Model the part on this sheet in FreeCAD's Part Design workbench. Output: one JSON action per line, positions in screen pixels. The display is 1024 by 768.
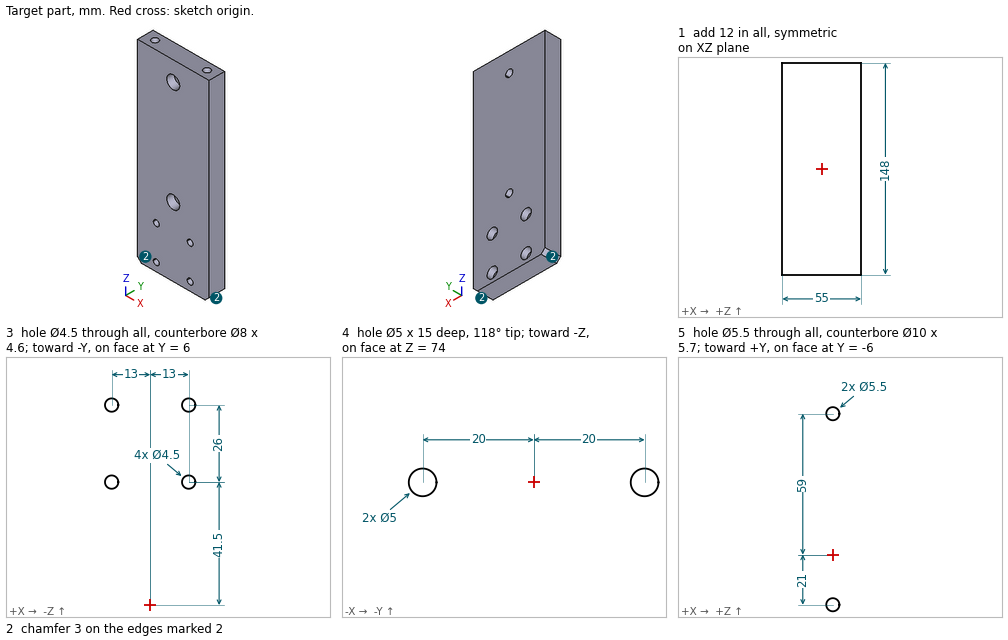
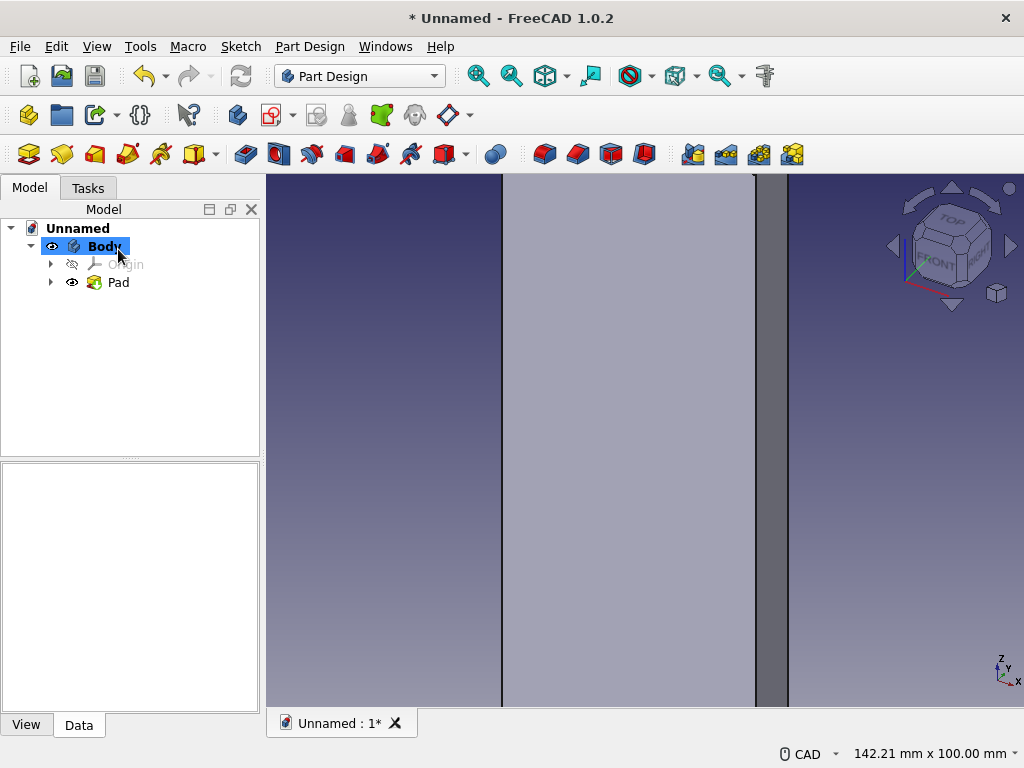
{"action": "key", "text": "v f"}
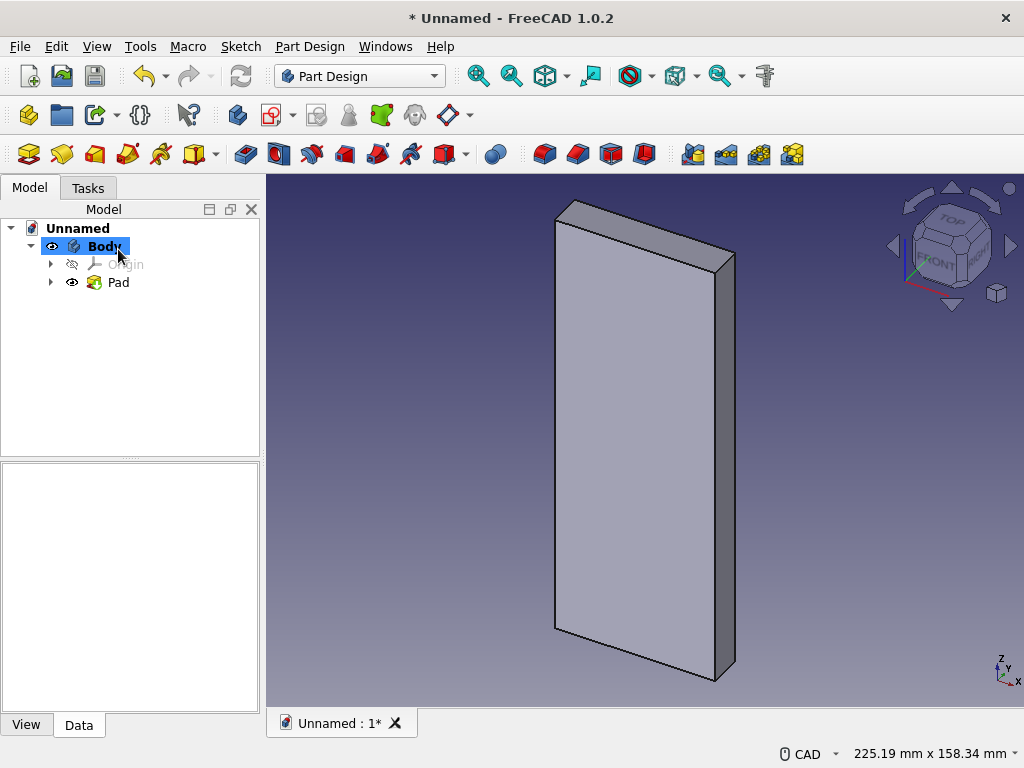
{"action": "key", "text": "0"}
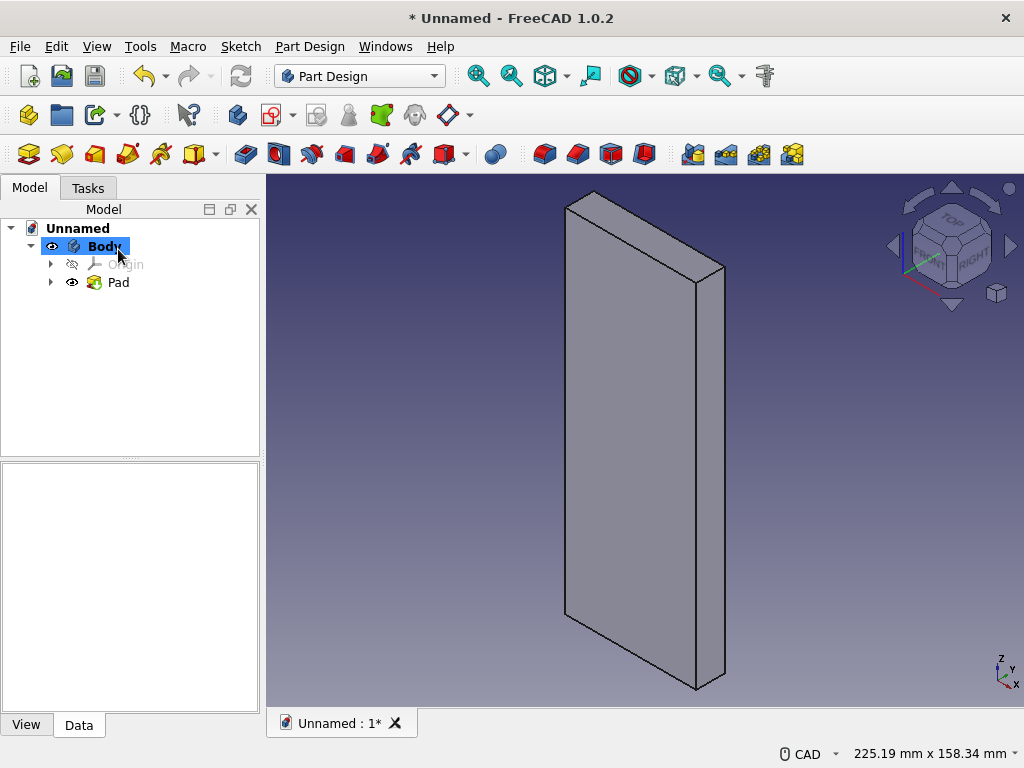
{"action": "key", "text": "2"}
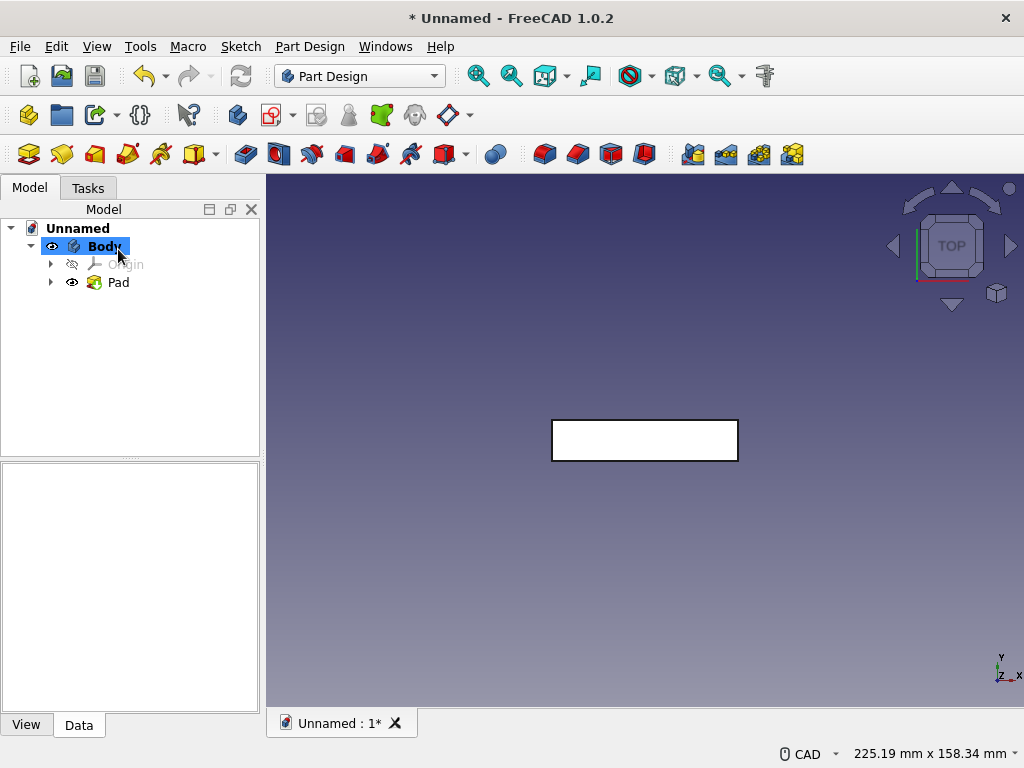
{"action": "key", "text": "v f"}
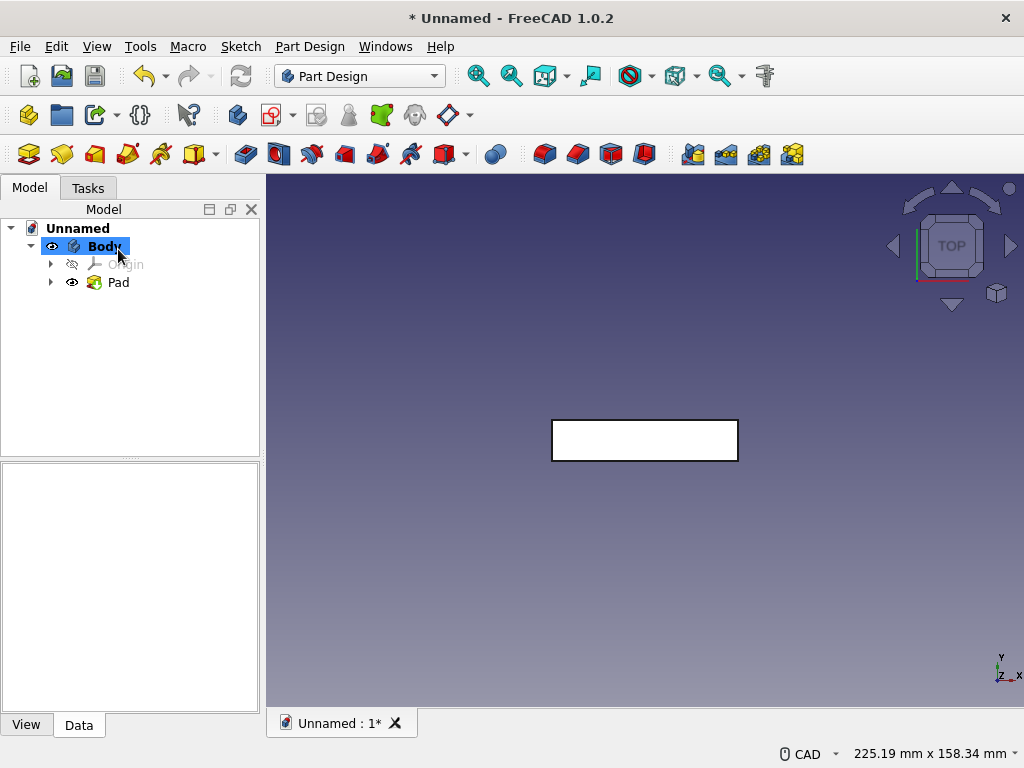
{"action": "key", "text": "1"}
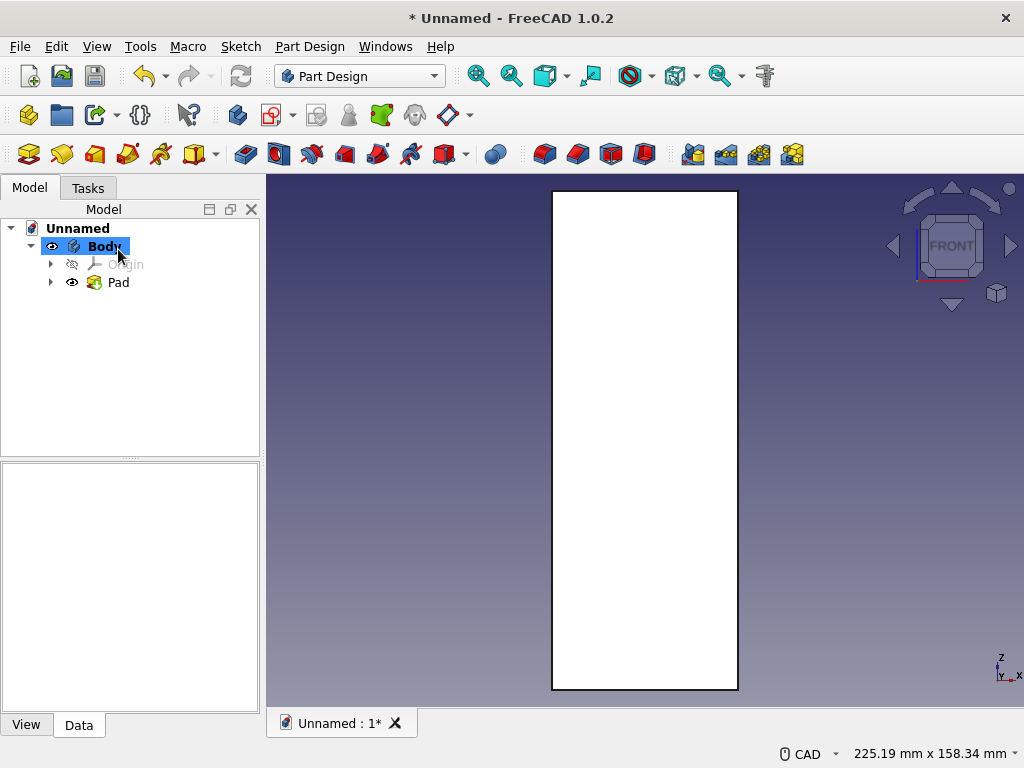
{"action": "key", "text": "3"}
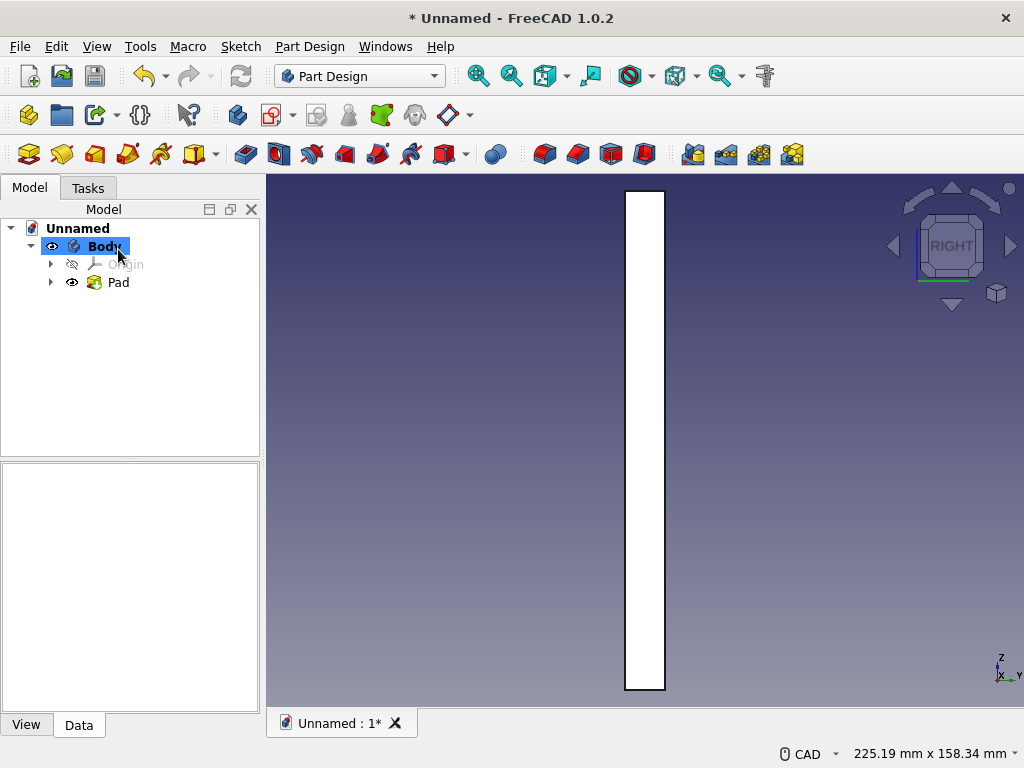
{"action": "key", "text": "5"}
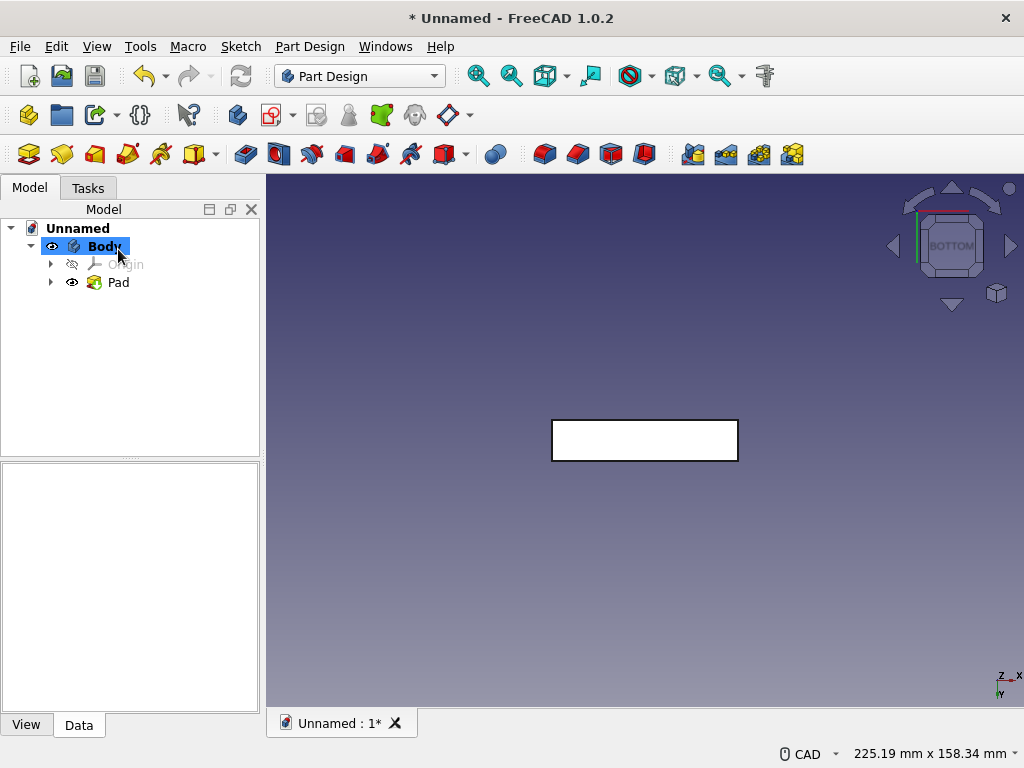
{"action": "key", "text": "v f"}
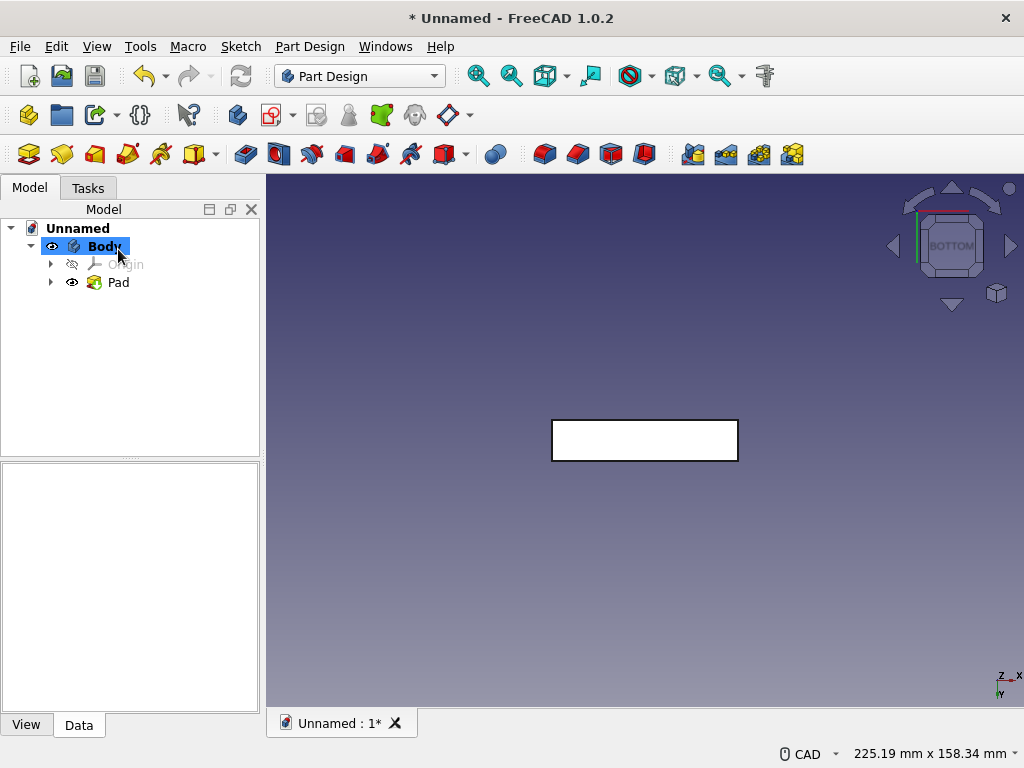
{"action": "left_click", "coordinate": [552, 439]}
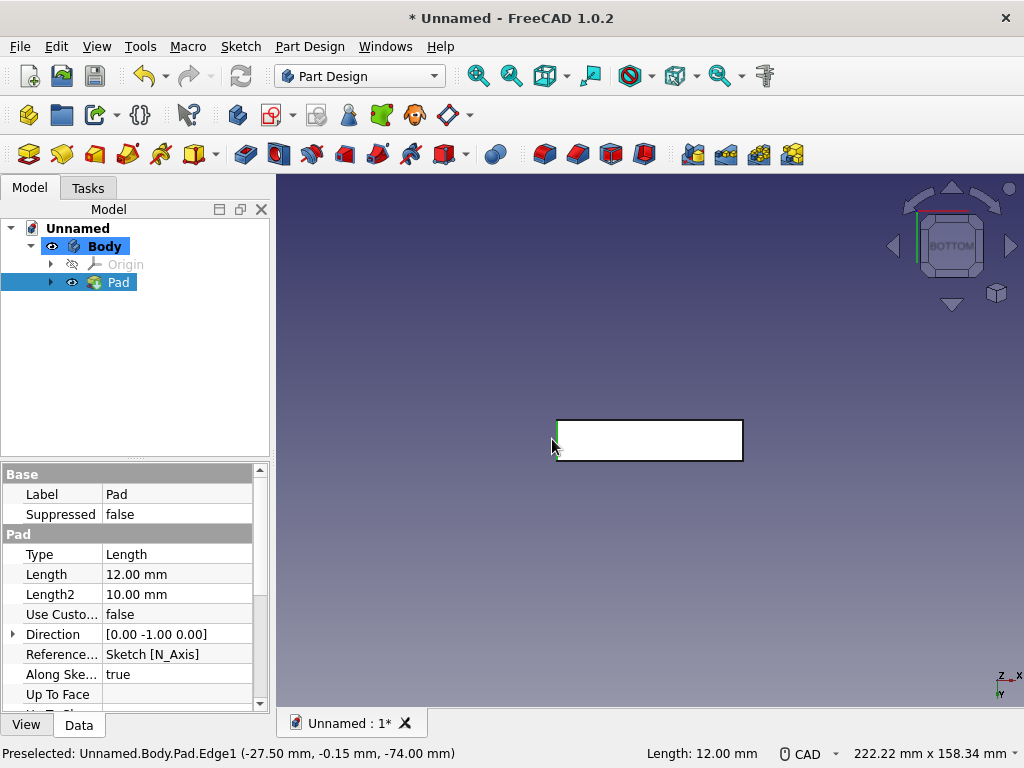
{"action": "left_click", "coordinate": [743, 439], "text": "ctrl"}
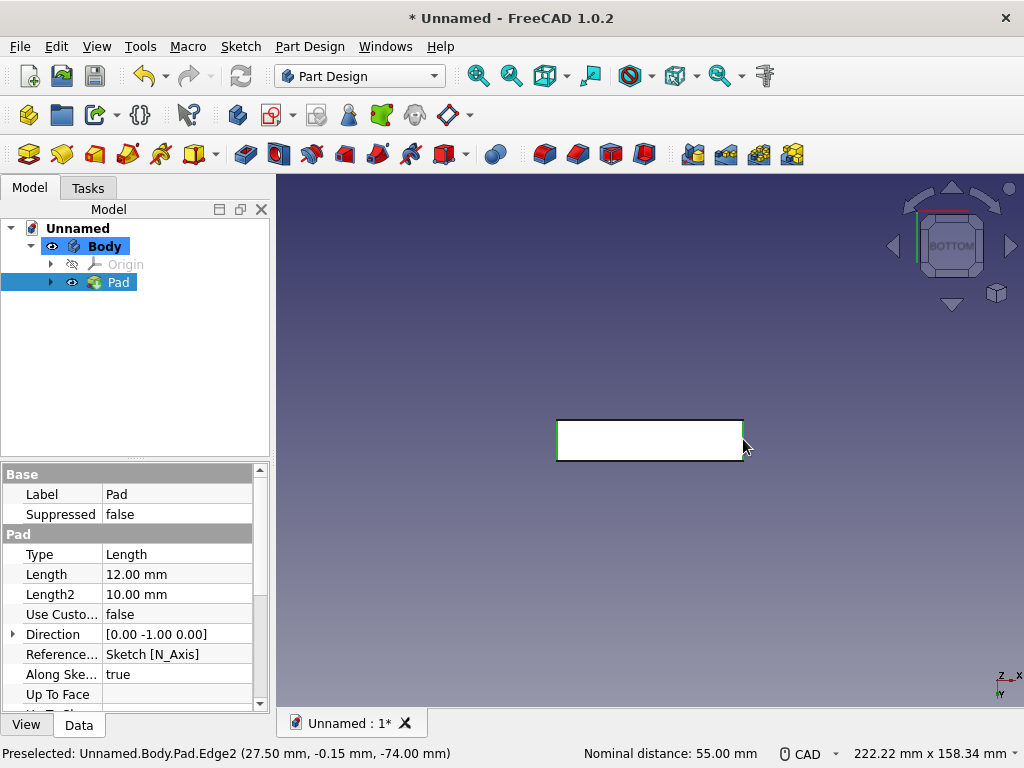
{"action": "left_click", "coordinate": [578, 154]}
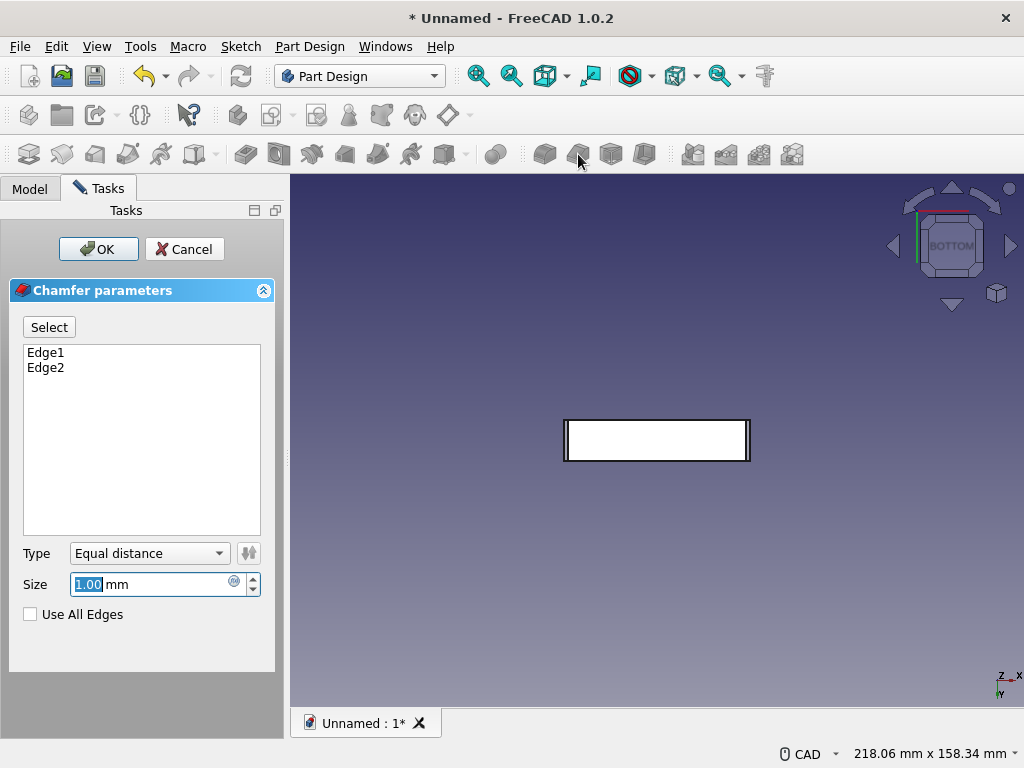
{"action": "type", "text": "3"}
{"action": "key", "text": "Tab"}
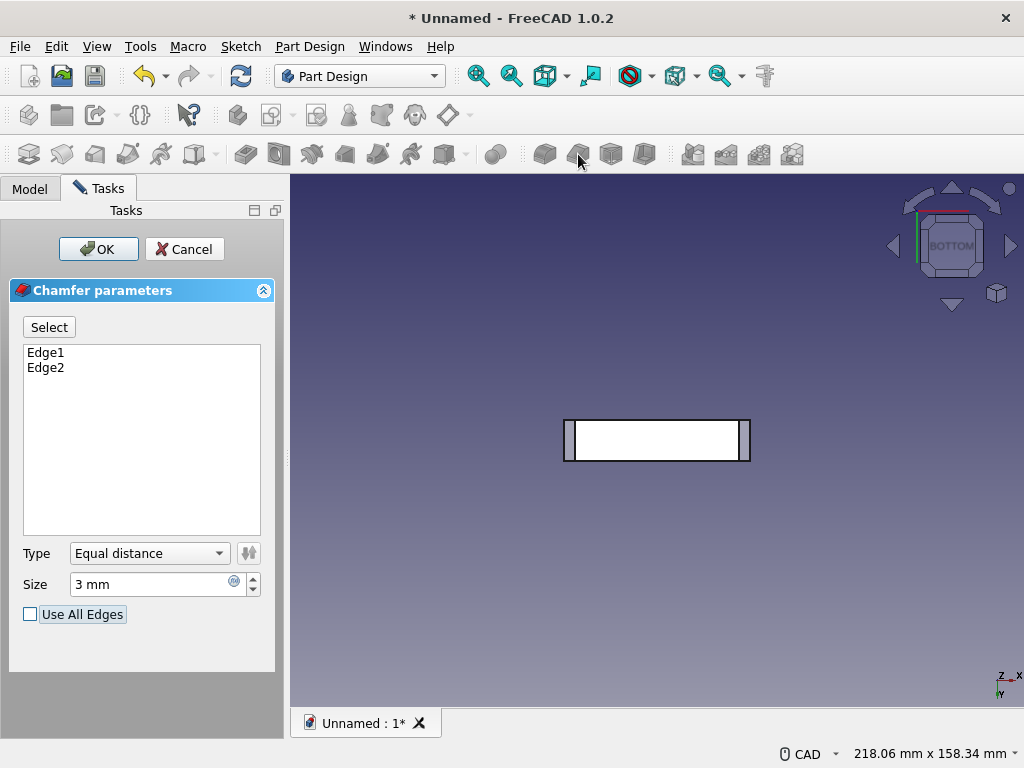
{"action": "left_click", "coordinate": [99, 249]}